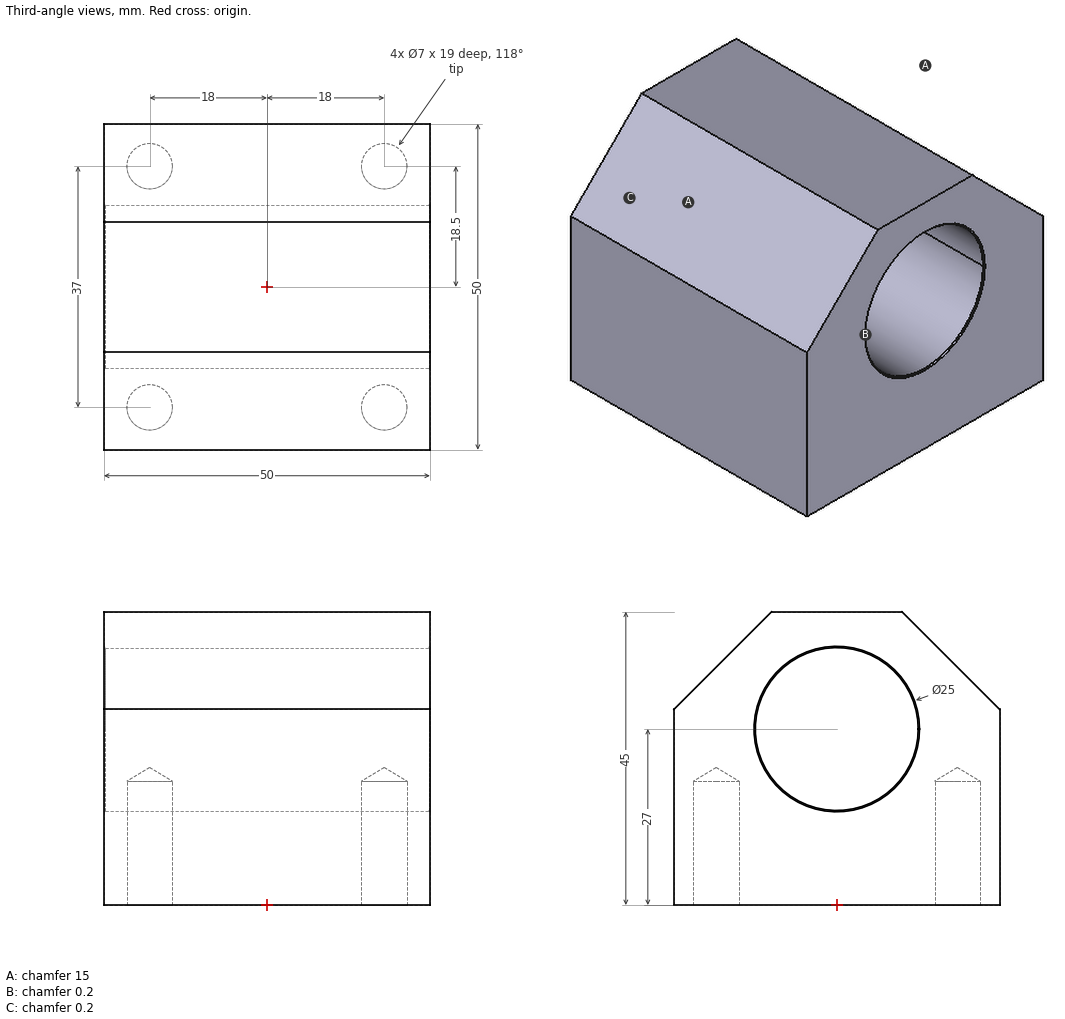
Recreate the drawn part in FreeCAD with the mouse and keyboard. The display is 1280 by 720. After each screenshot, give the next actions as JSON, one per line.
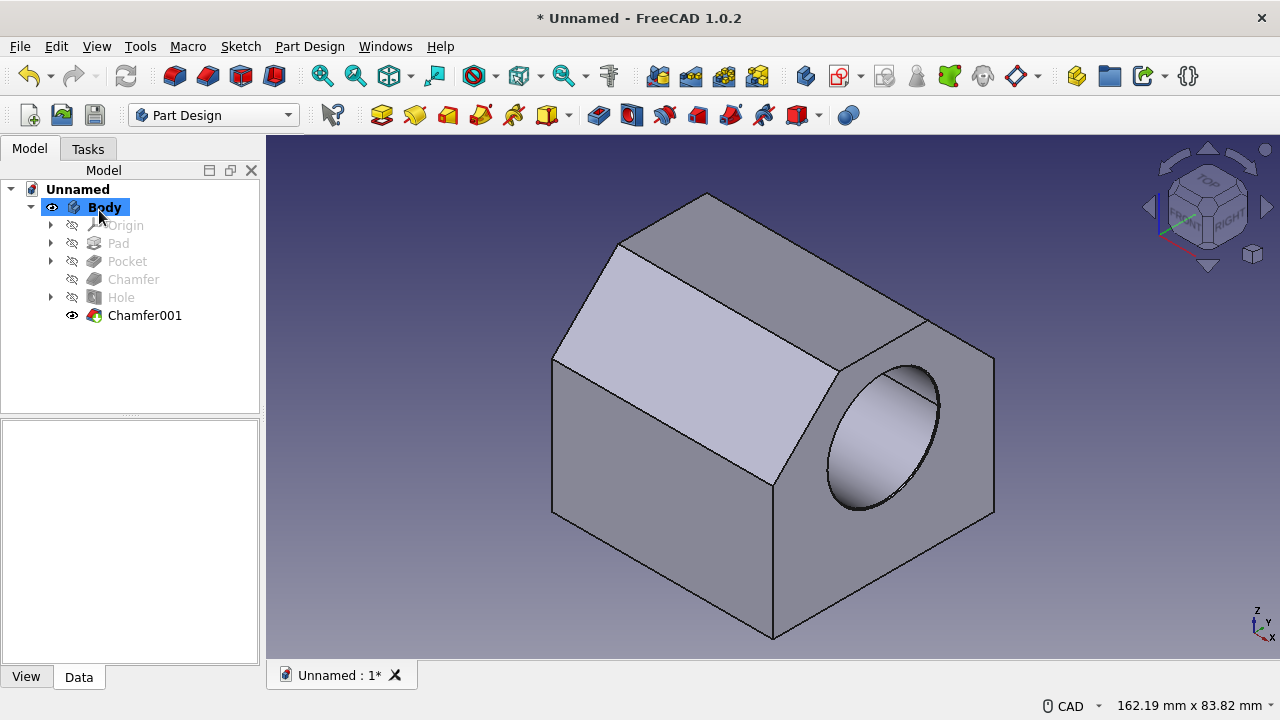
{"action": "key", "text": "1"}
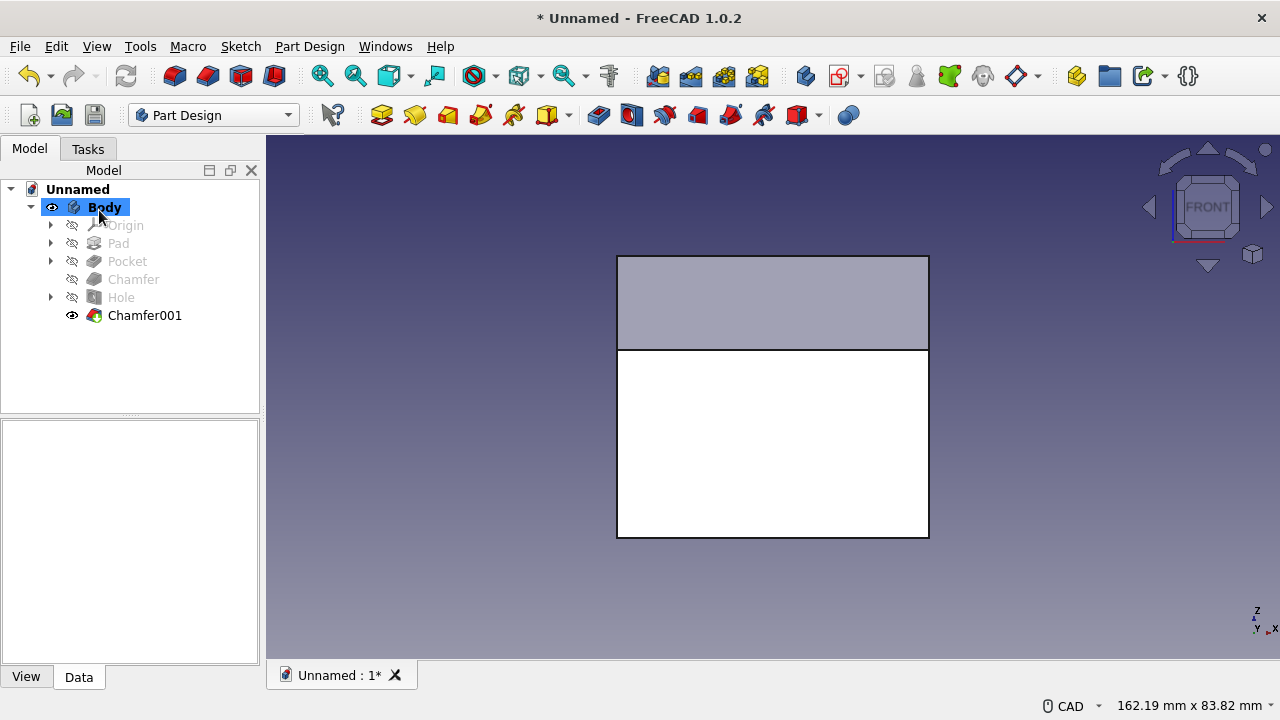
{"action": "key", "text": "3"}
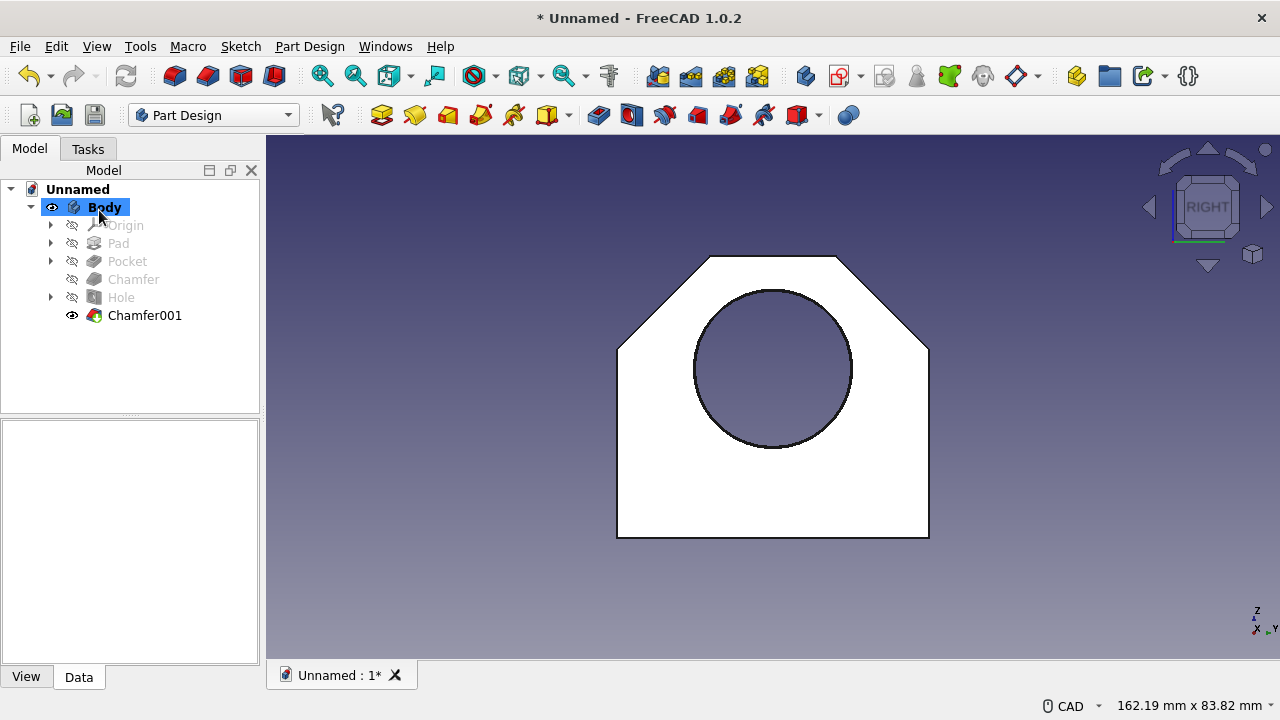
{"action": "key", "text": "5"}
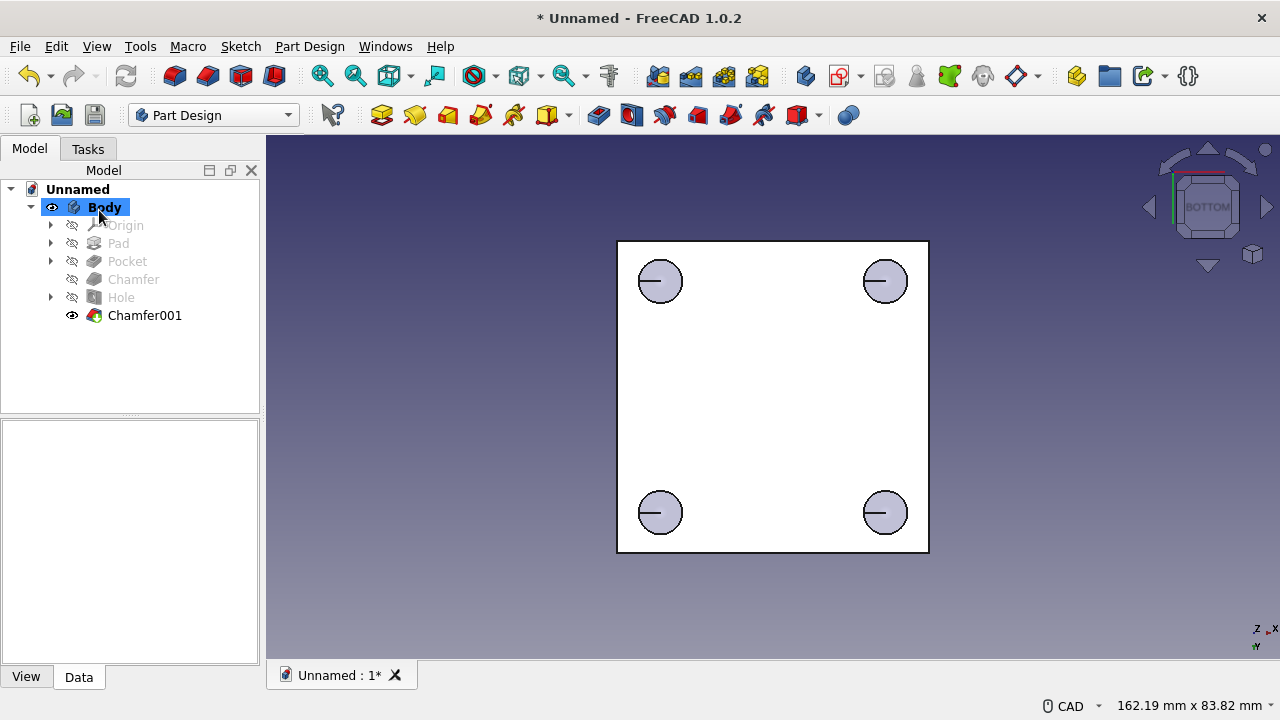
{"action": "key", "text": "4"}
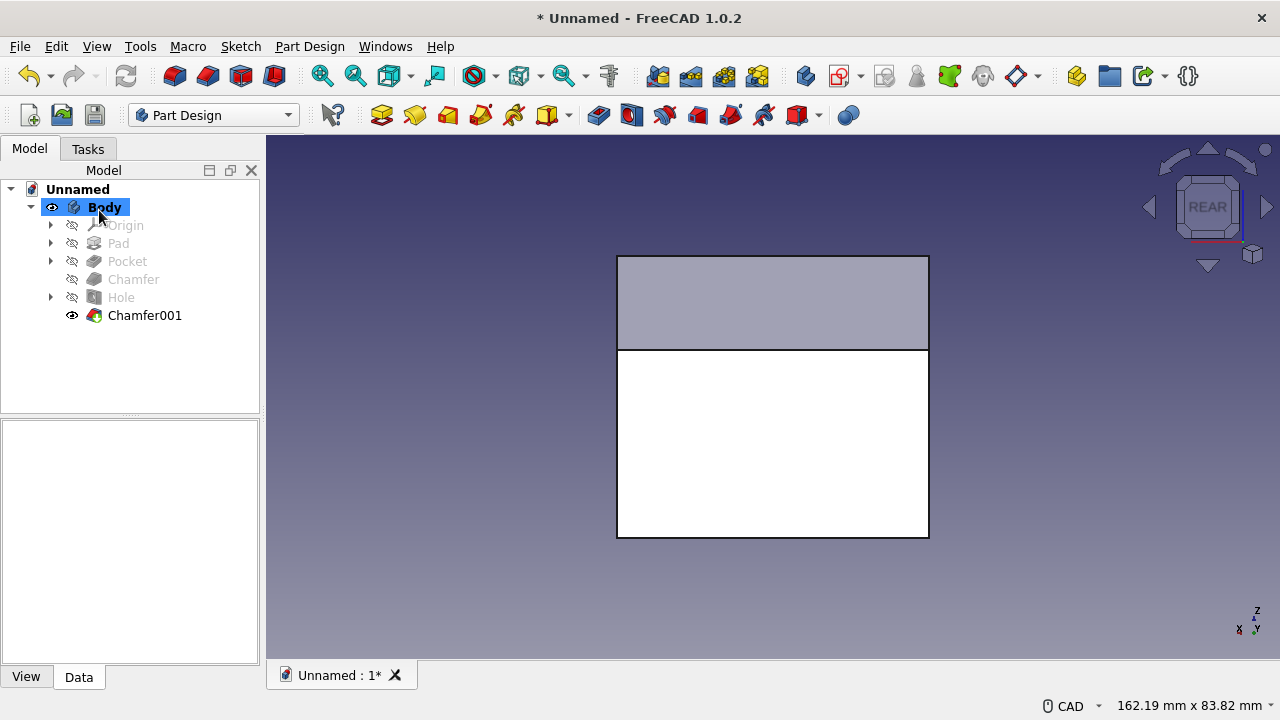
{"action": "key", "text": "6"}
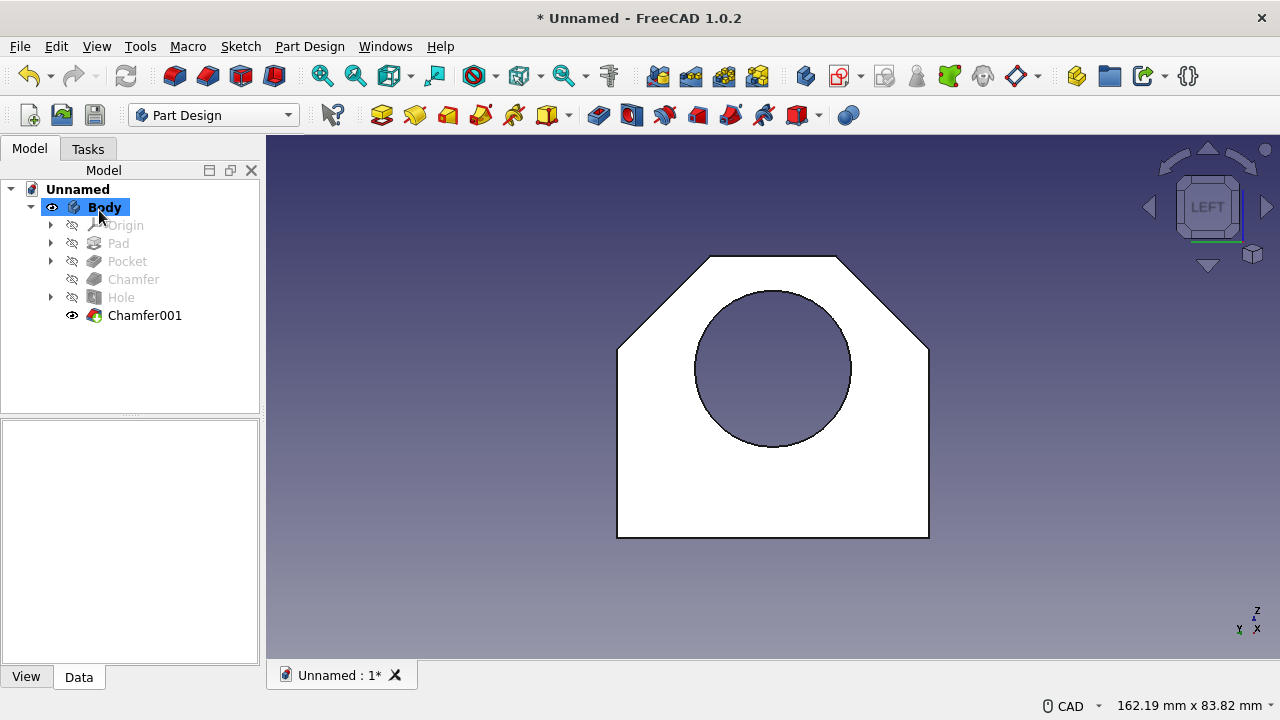
{"action": "left_click", "coordinate": [851, 368]}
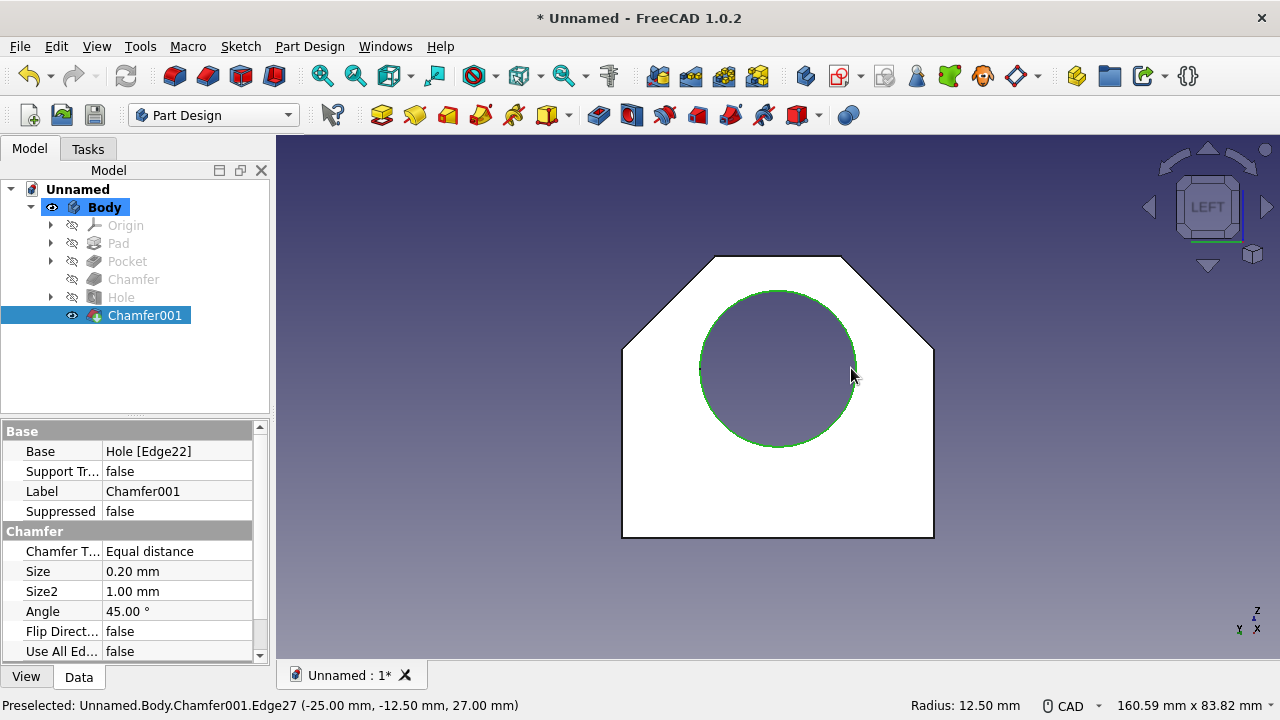
{"action": "left_click", "coordinate": [208, 76]}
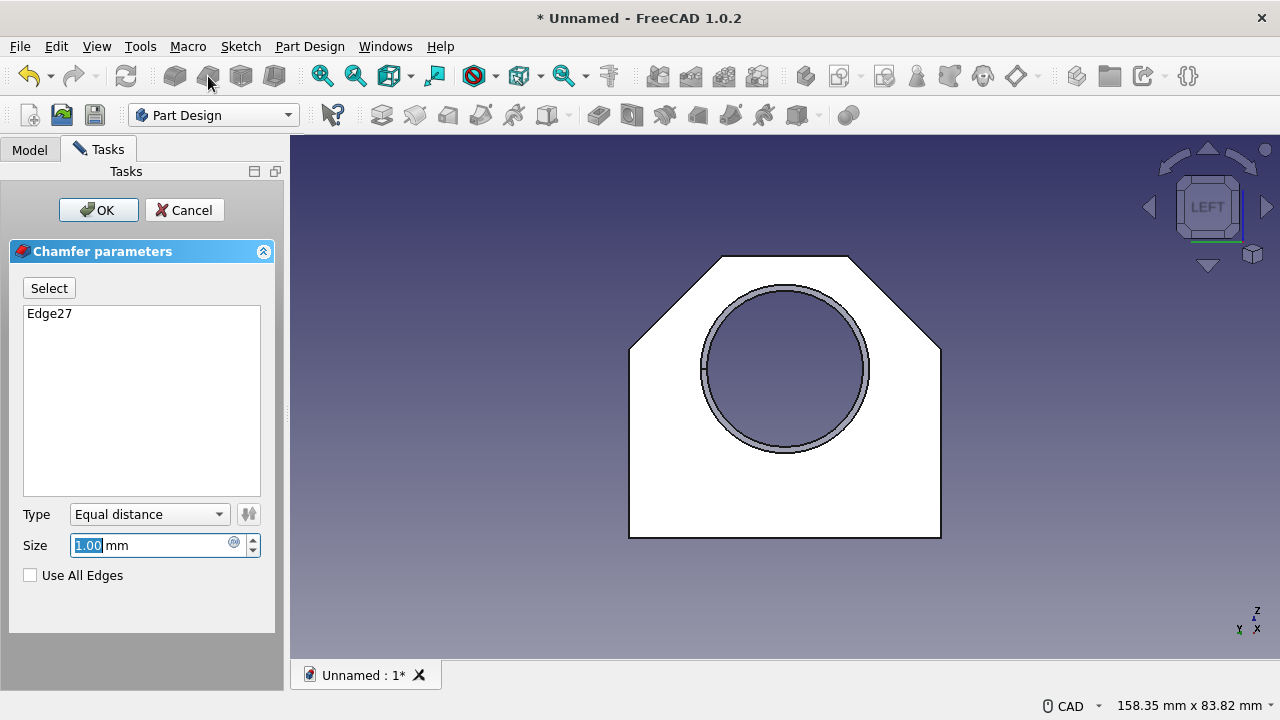
{"action": "type", "text": "0.2"}
{"action": "key", "text": "Tab"}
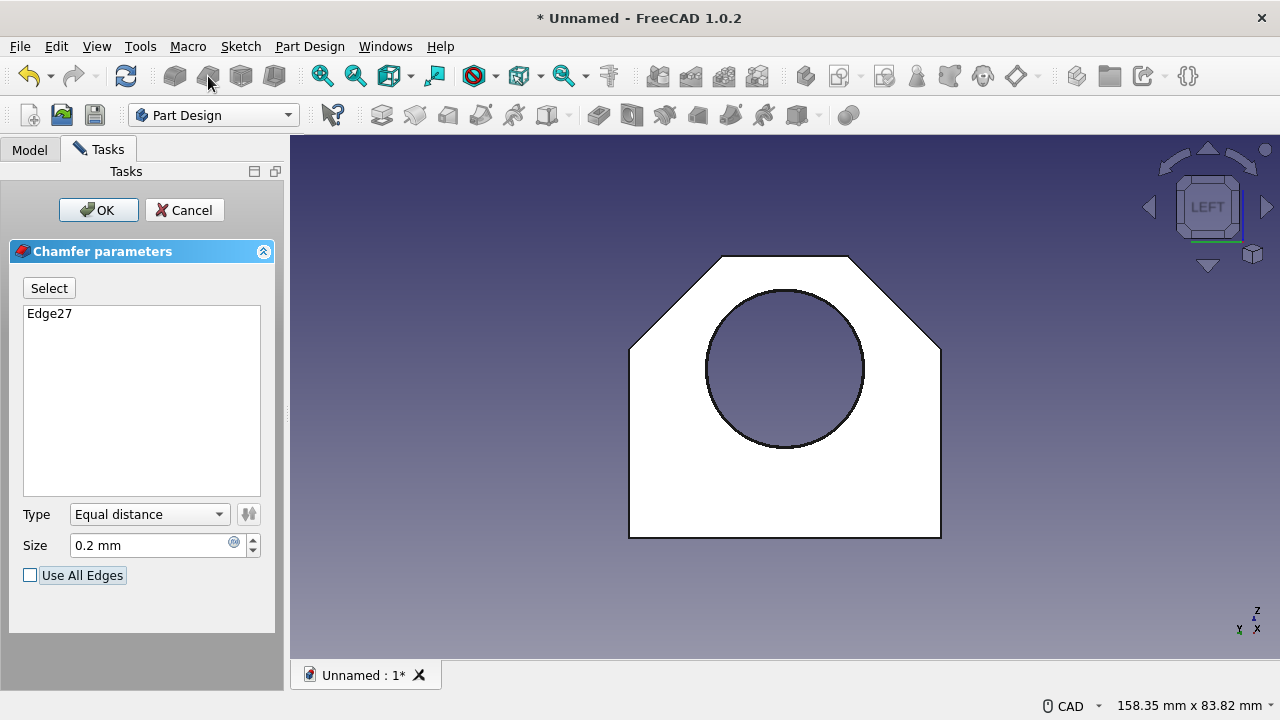
{"action": "left_click", "coordinate": [99, 210]}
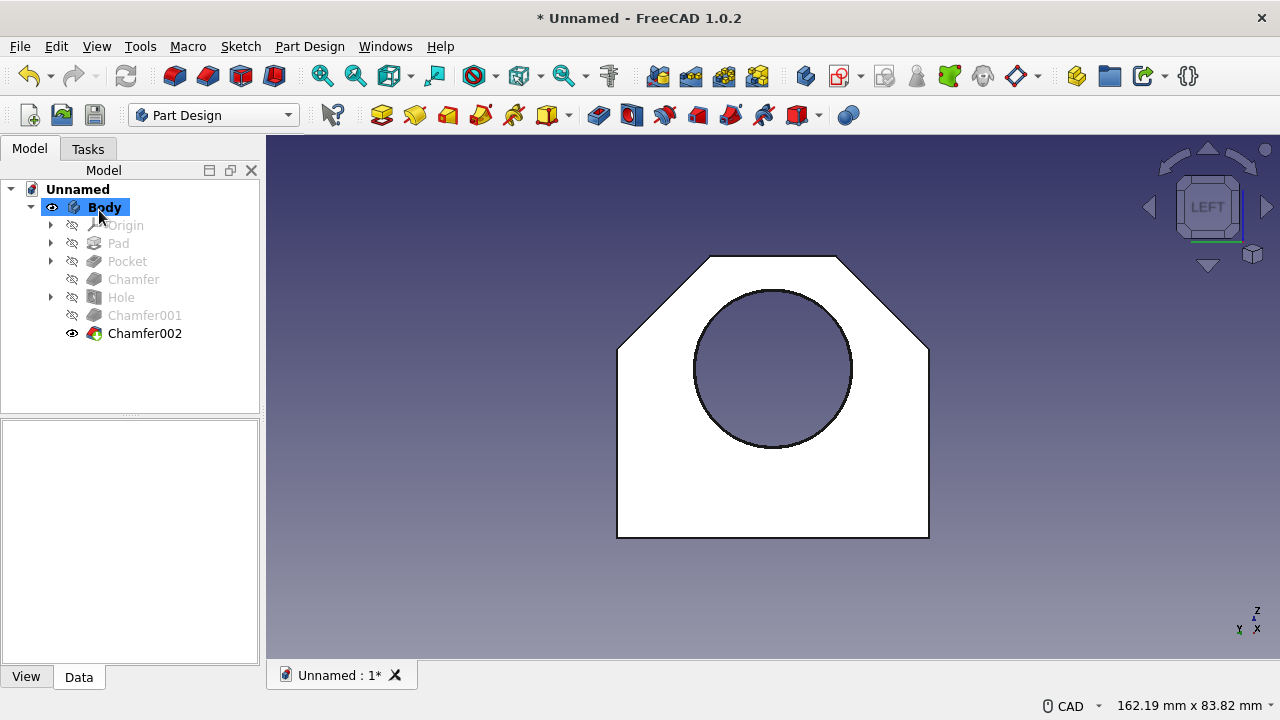
{"action": "key", "text": "0"}